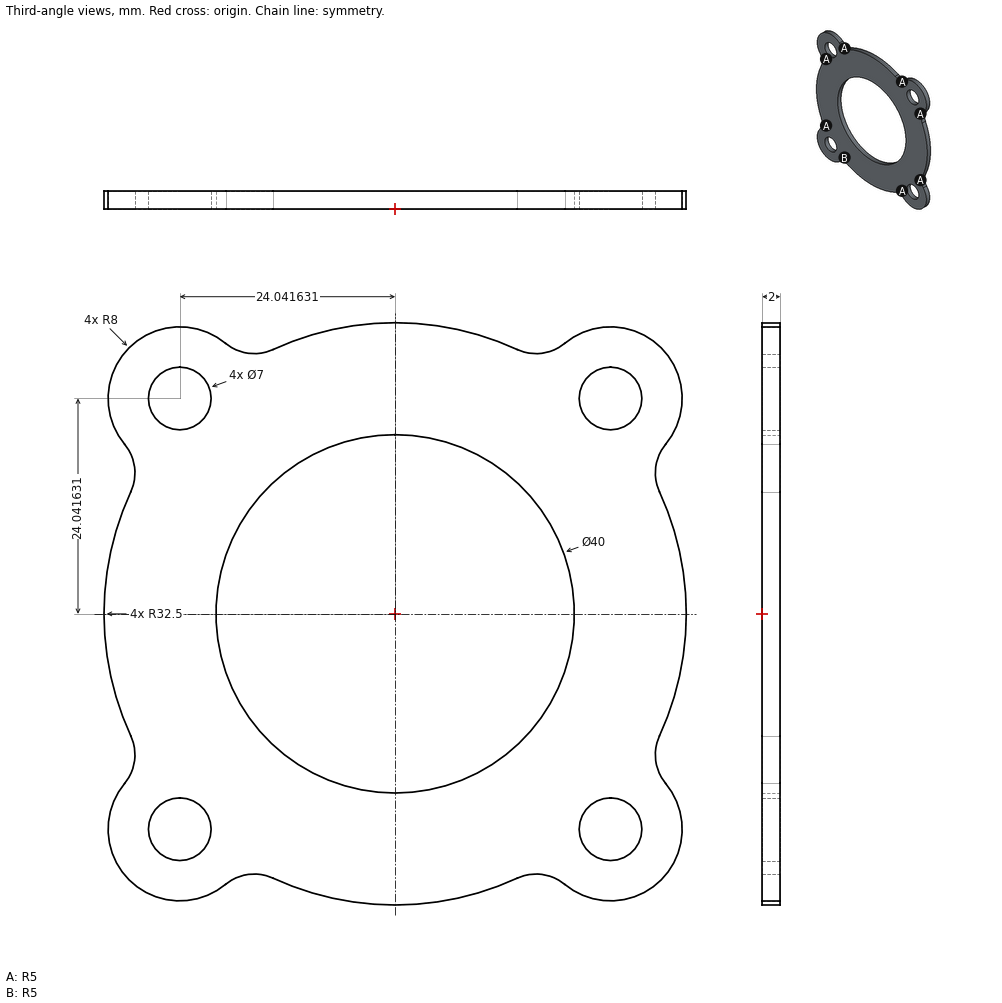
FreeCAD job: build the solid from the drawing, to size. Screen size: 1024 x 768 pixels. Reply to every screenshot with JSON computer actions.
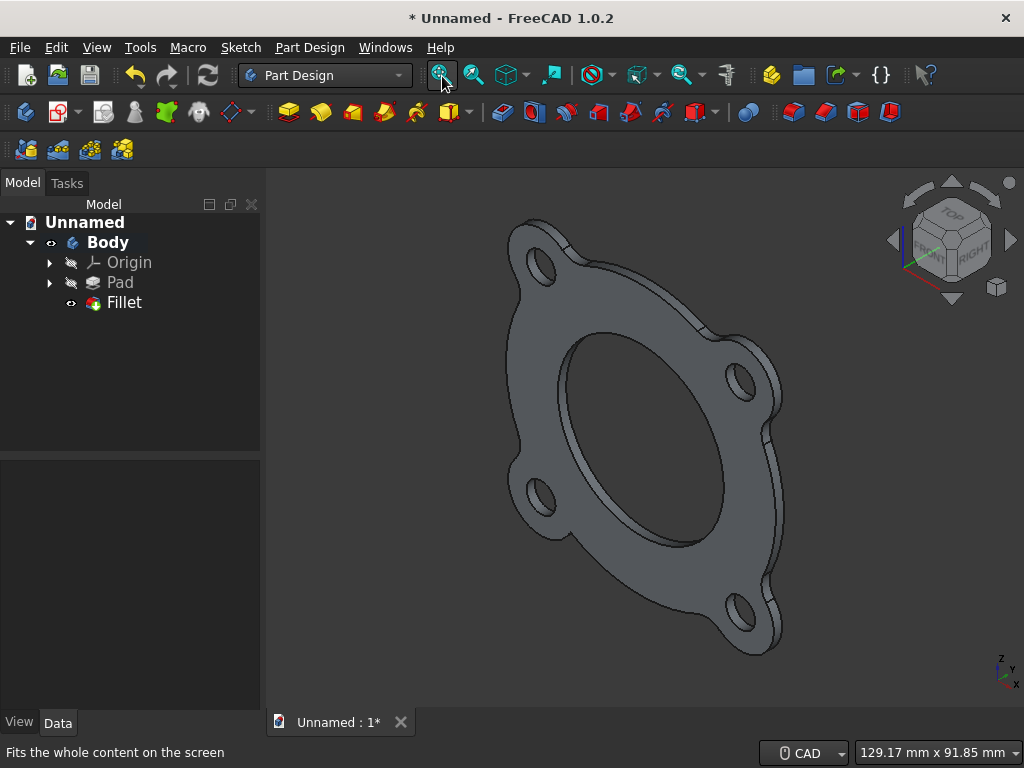
{"action": "key", "text": "2"}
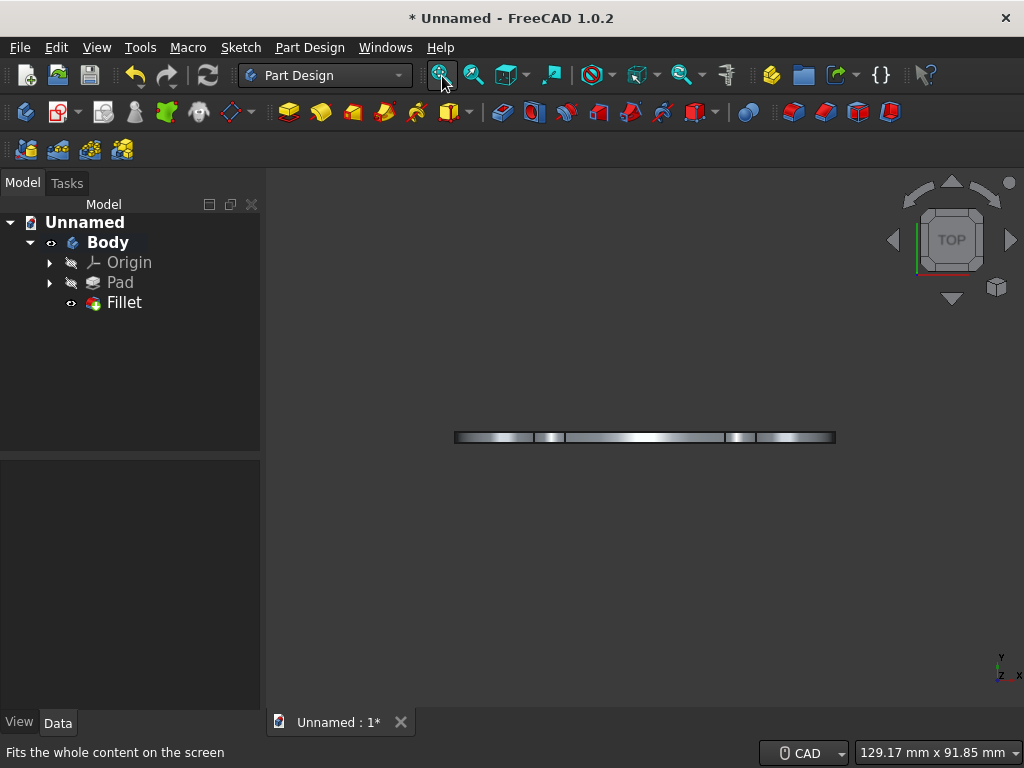
{"action": "scroll", "coordinate": [546, 436], "scroll_direction": "up", "scroll_amount": 7}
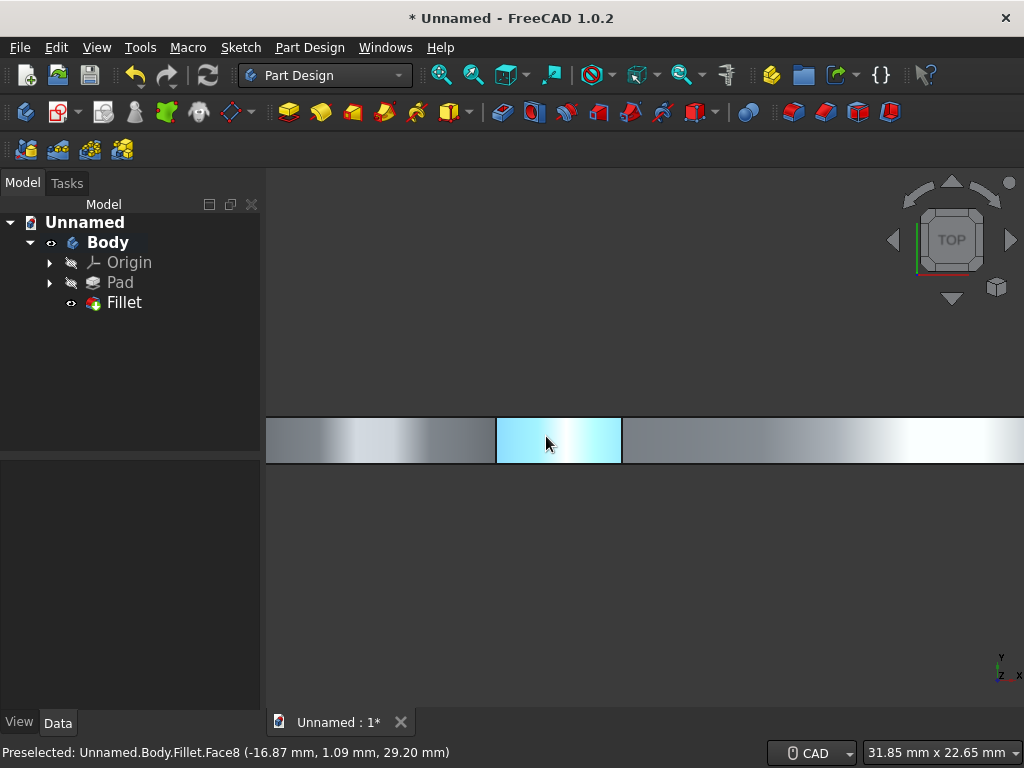
{"action": "key", "text": "v f"}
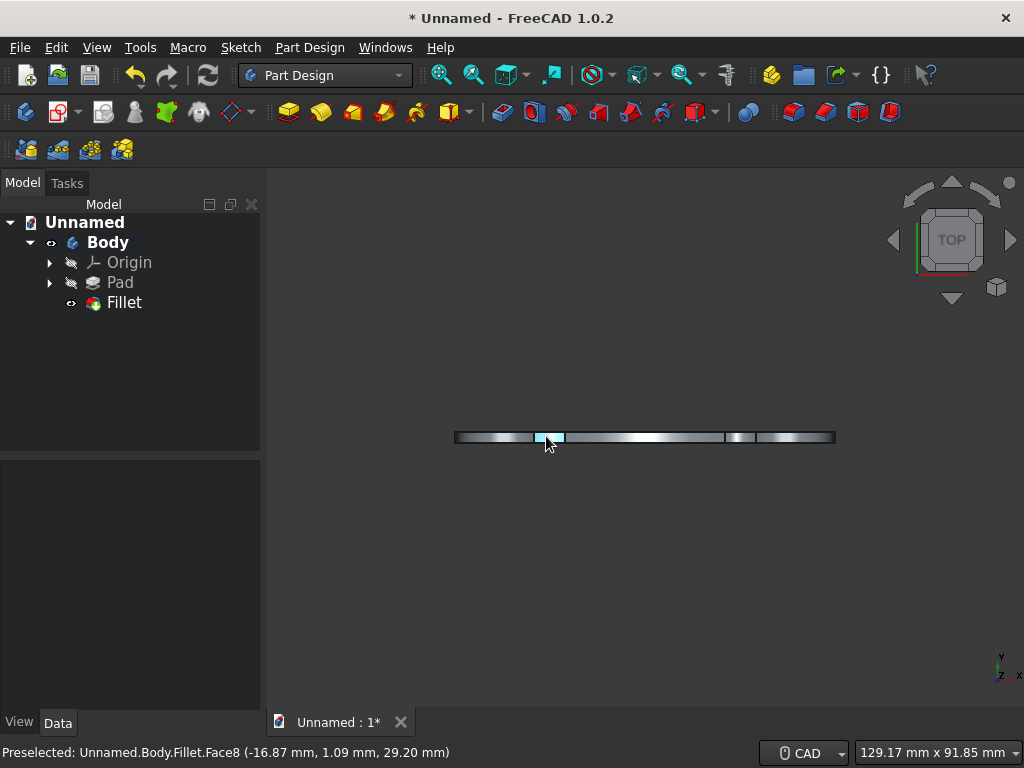
{"action": "key", "text": "1"}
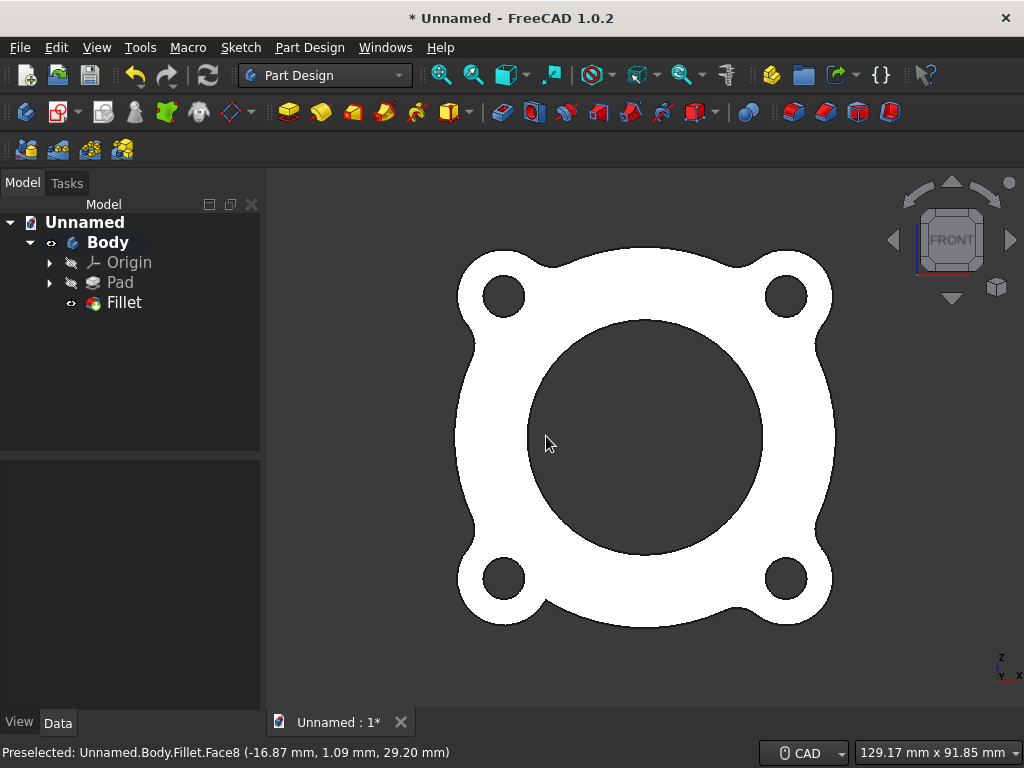
{"action": "scroll", "coordinate": [546, 599], "scroll_direction": "up", "scroll_amount": 7}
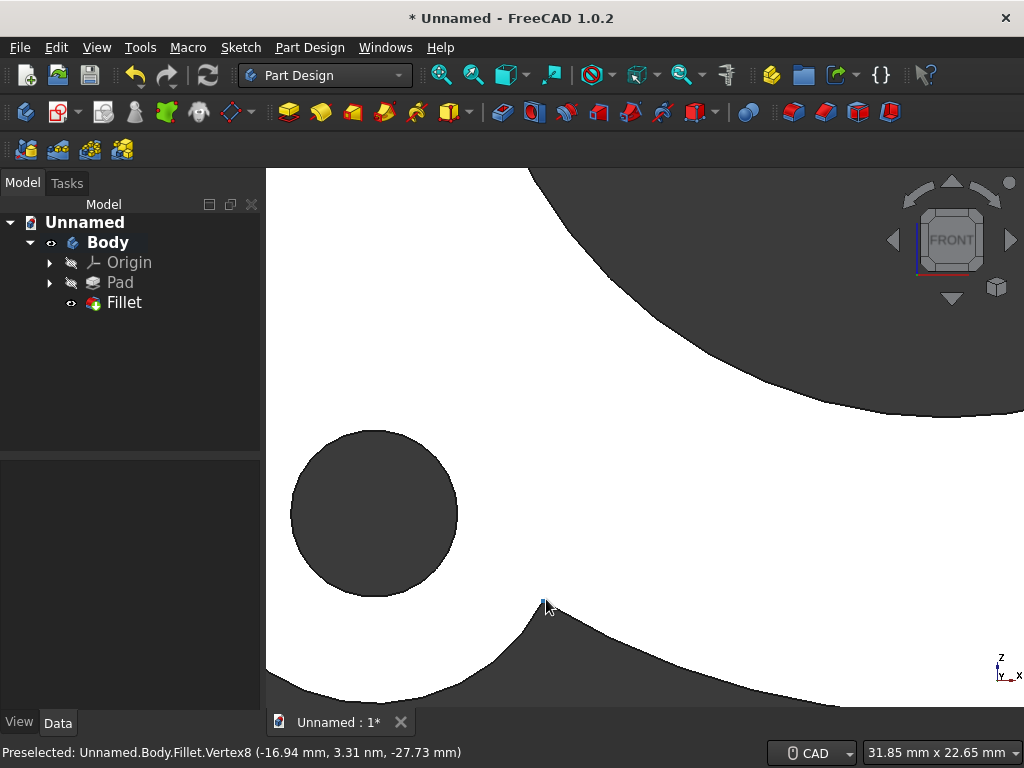
{"action": "left_click", "coordinate": [442, 76]}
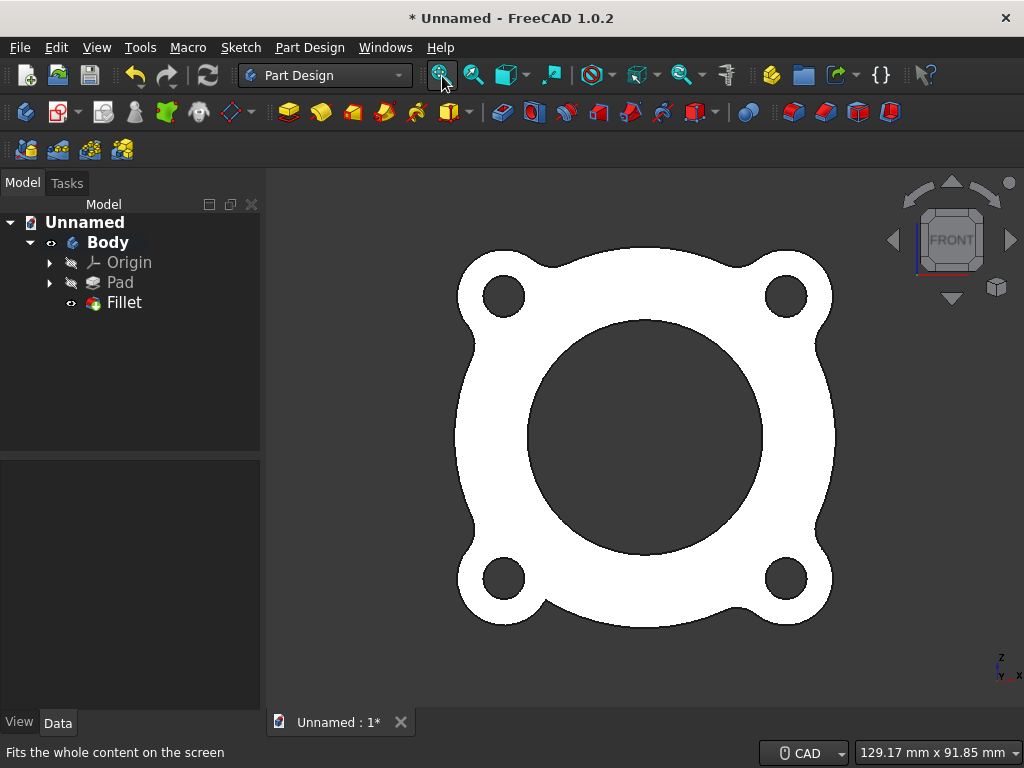
{"action": "key", "text": "3"}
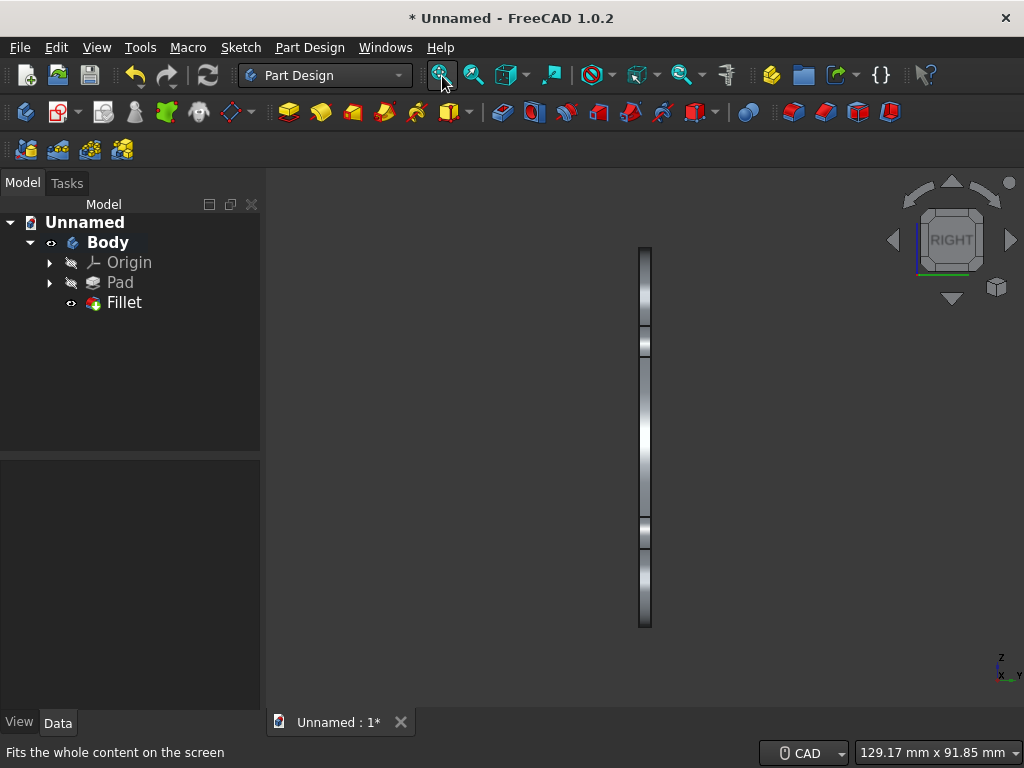
{"action": "scroll", "coordinate": [645, 599], "scroll_direction": "up", "scroll_amount": 7}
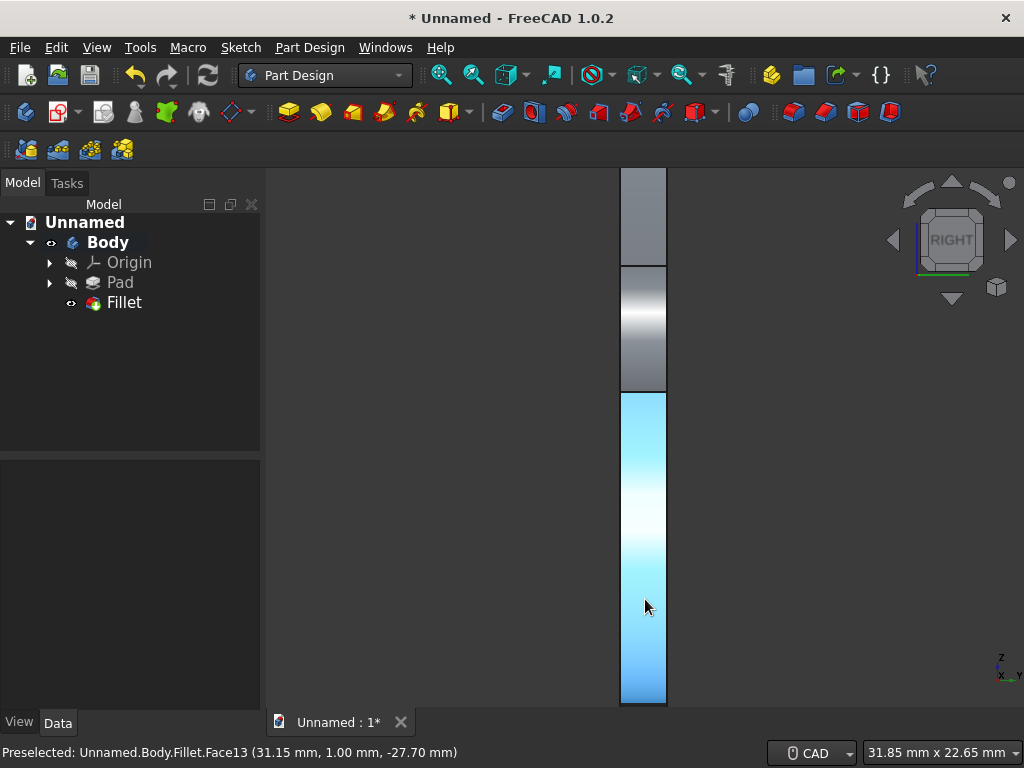
{"action": "left_click", "coordinate": [442, 76]}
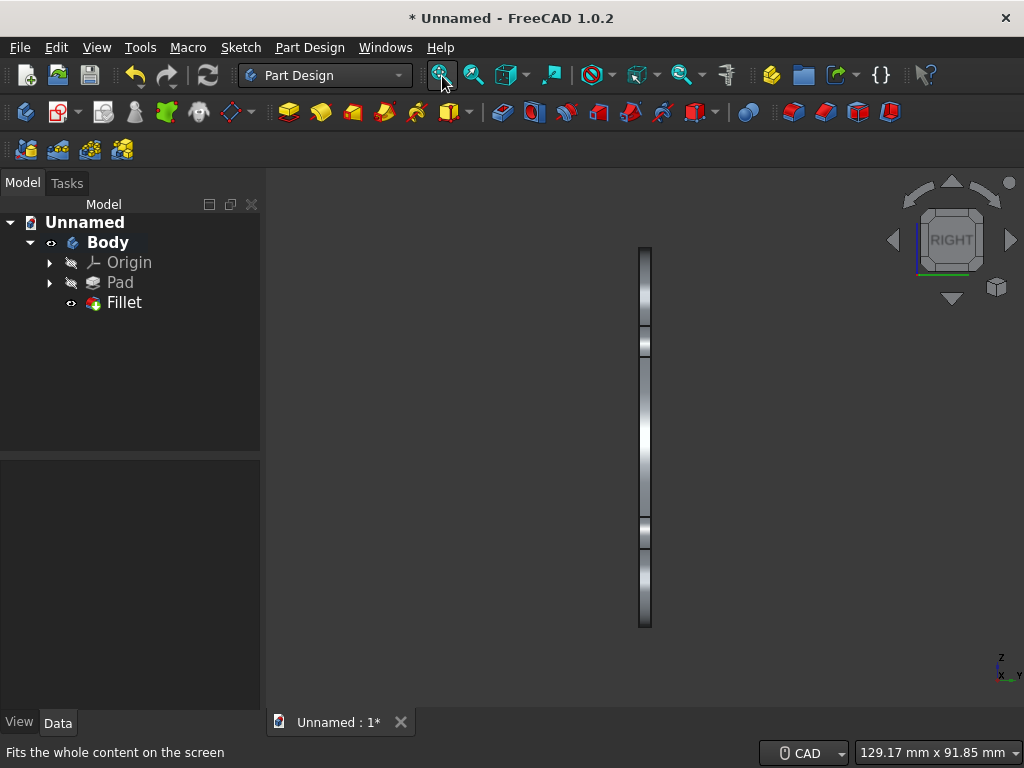
{"action": "key", "text": "5"}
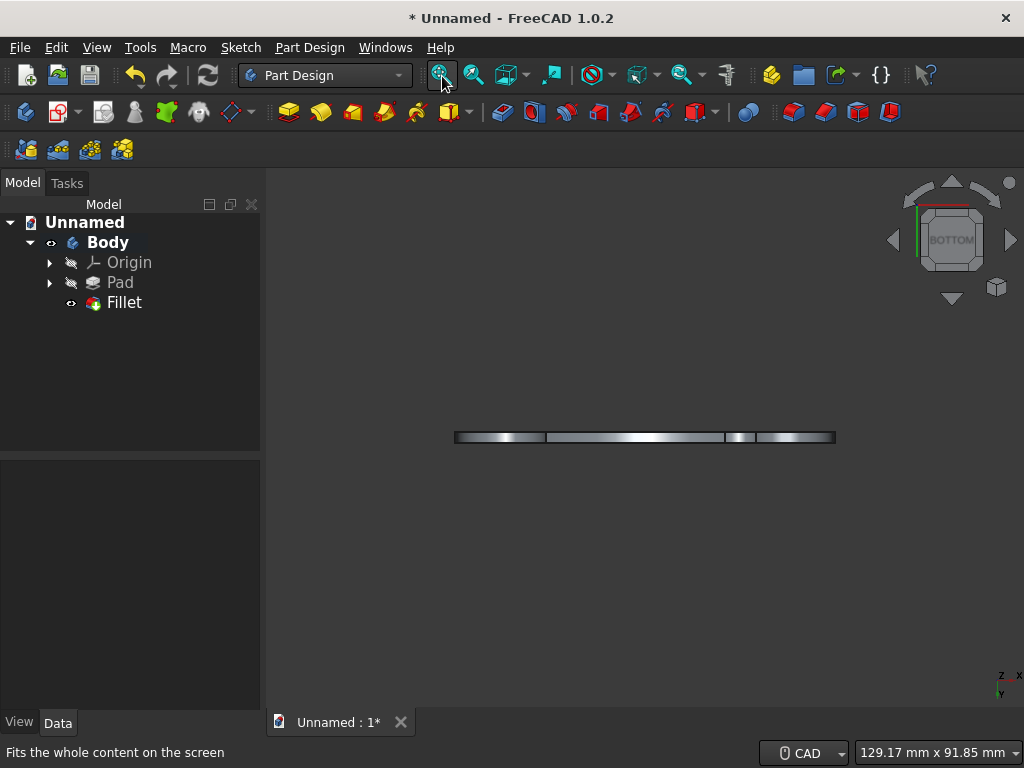
{"action": "scroll", "coordinate": [546, 436], "scroll_direction": "up", "scroll_amount": 7}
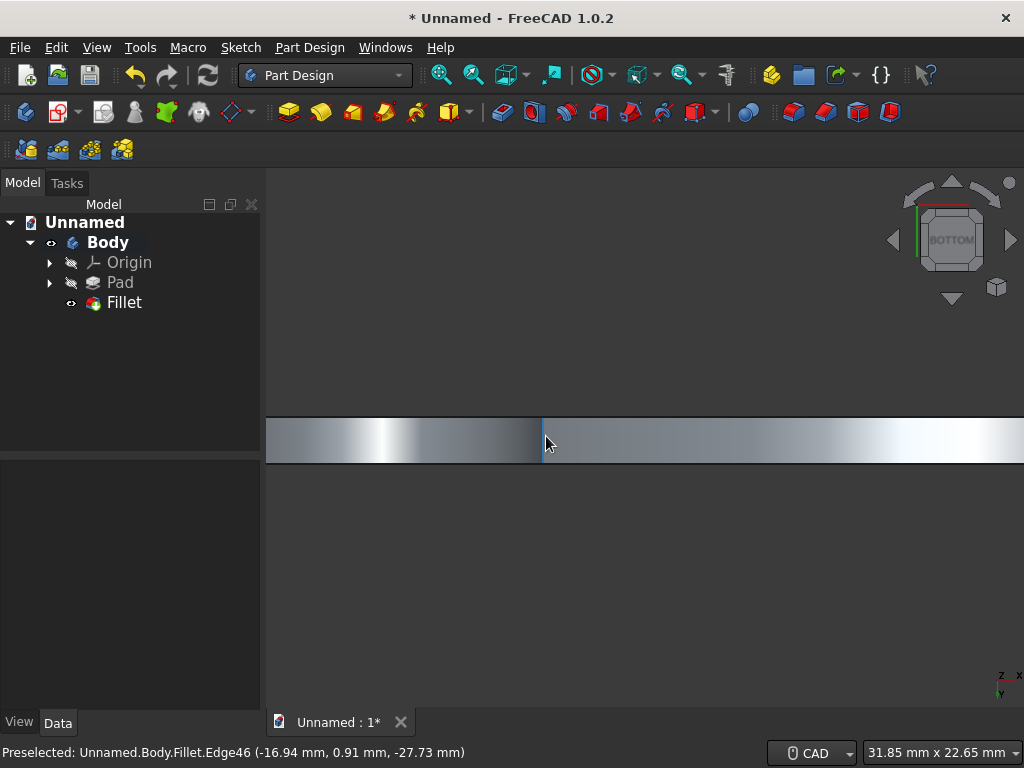
{"action": "left_click", "coordinate": [442, 76]}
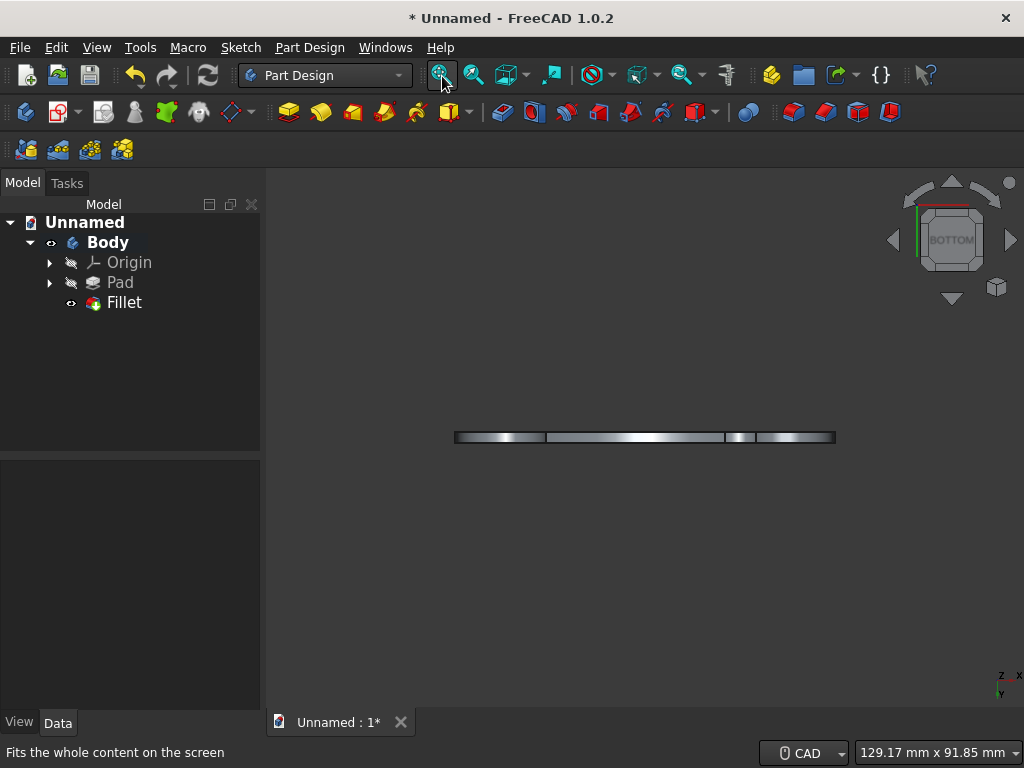
{"action": "key", "text": "4"}